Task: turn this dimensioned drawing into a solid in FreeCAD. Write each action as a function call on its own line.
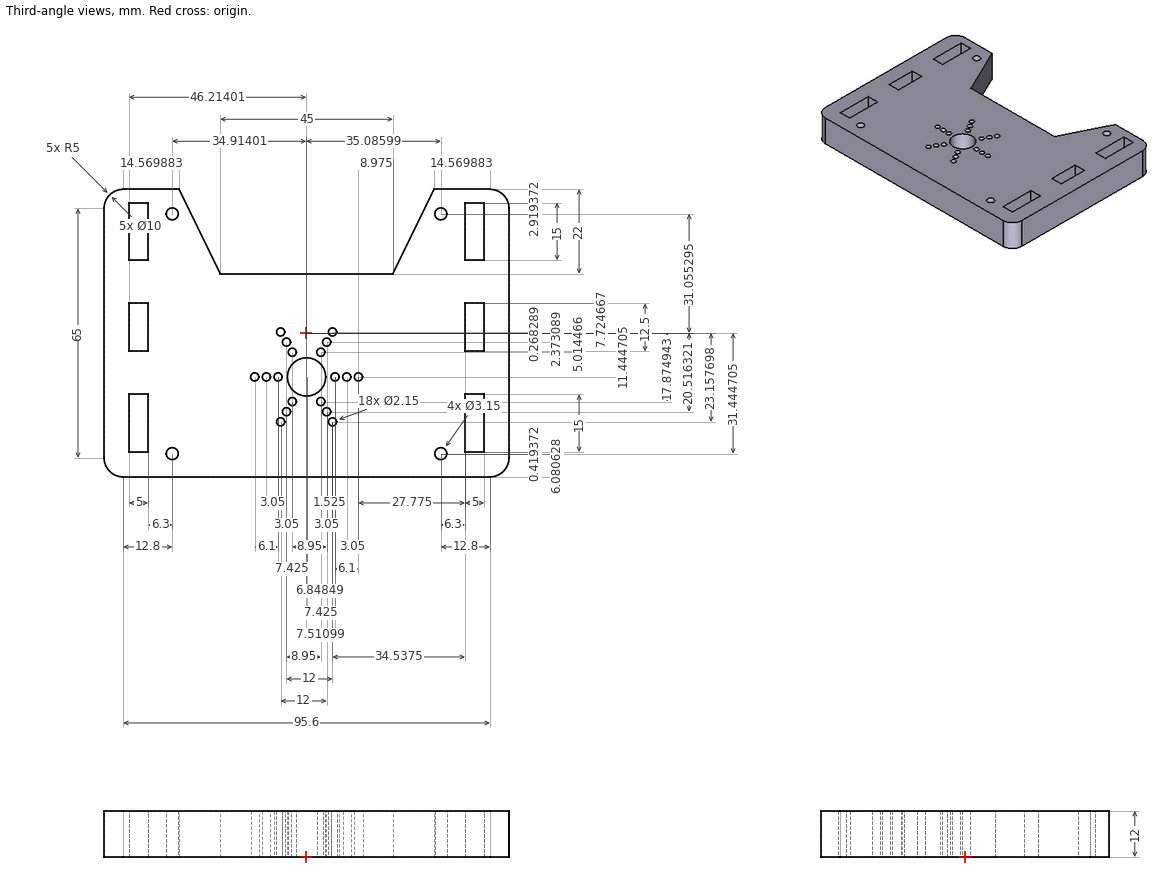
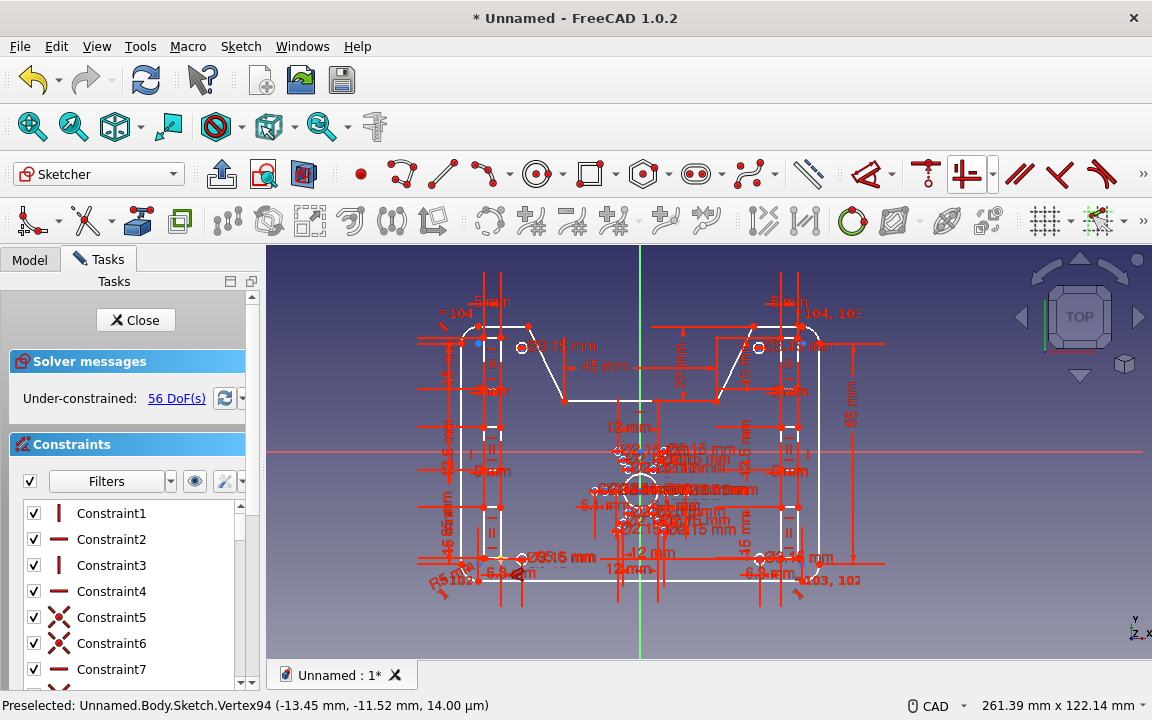
scroll(781, 338, up, 4)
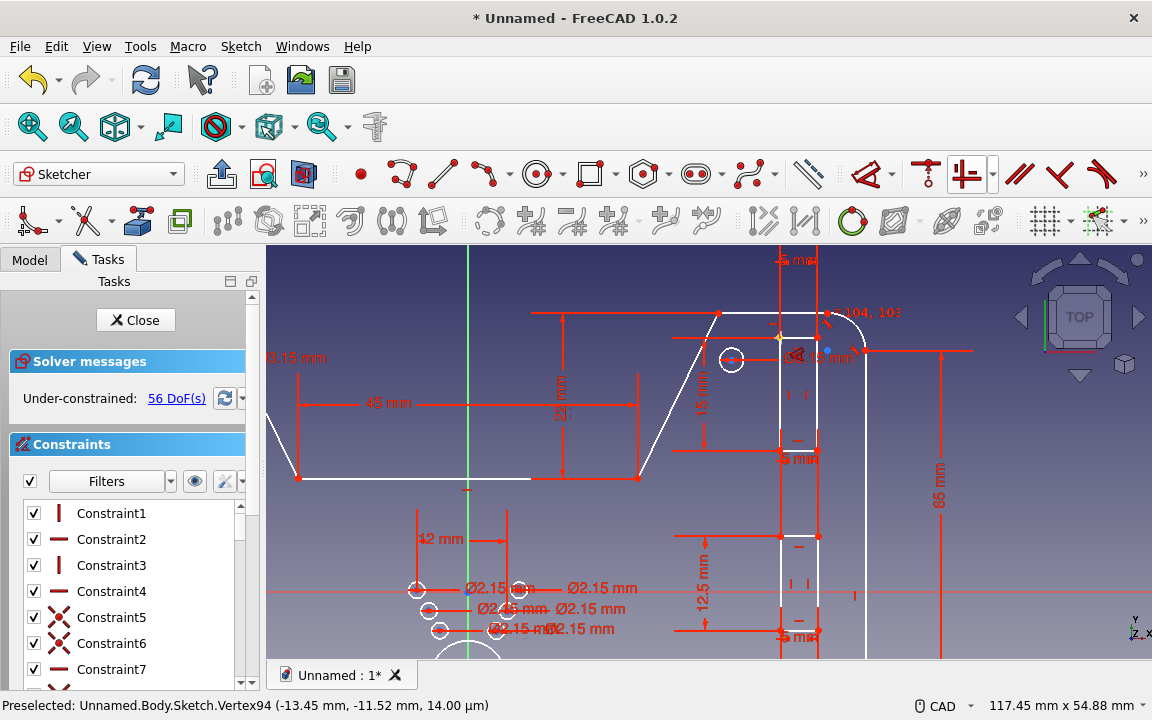
click(780, 338)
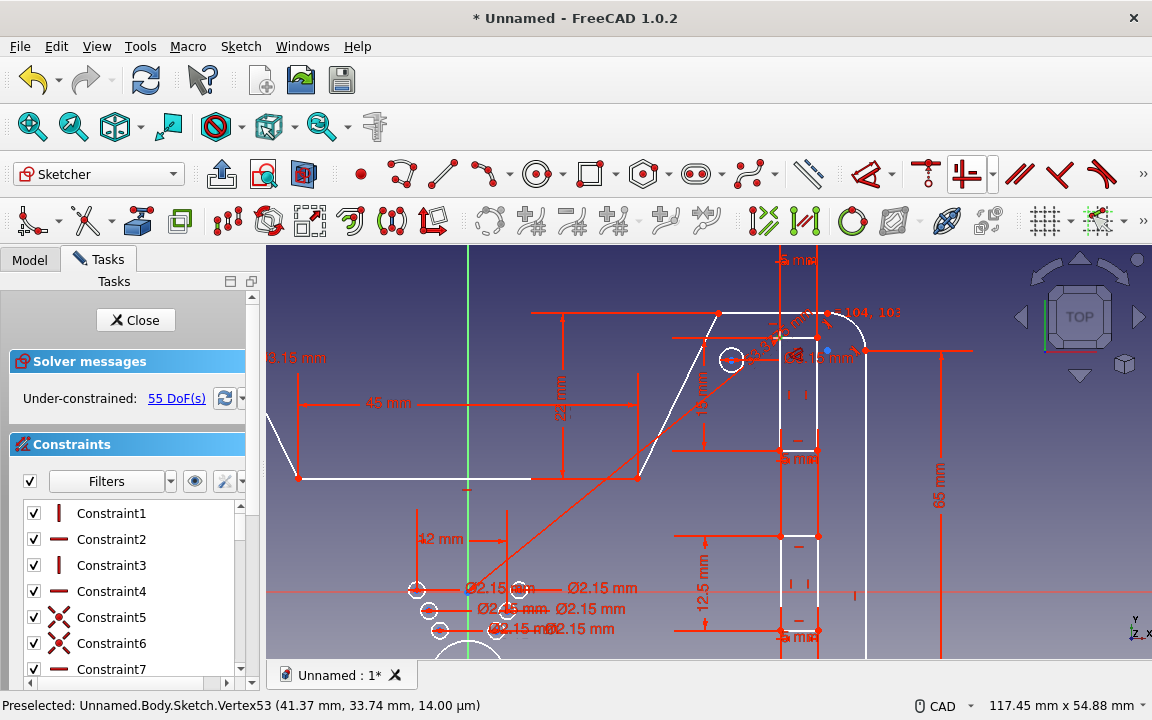
click(732, 360)
click(756, 394)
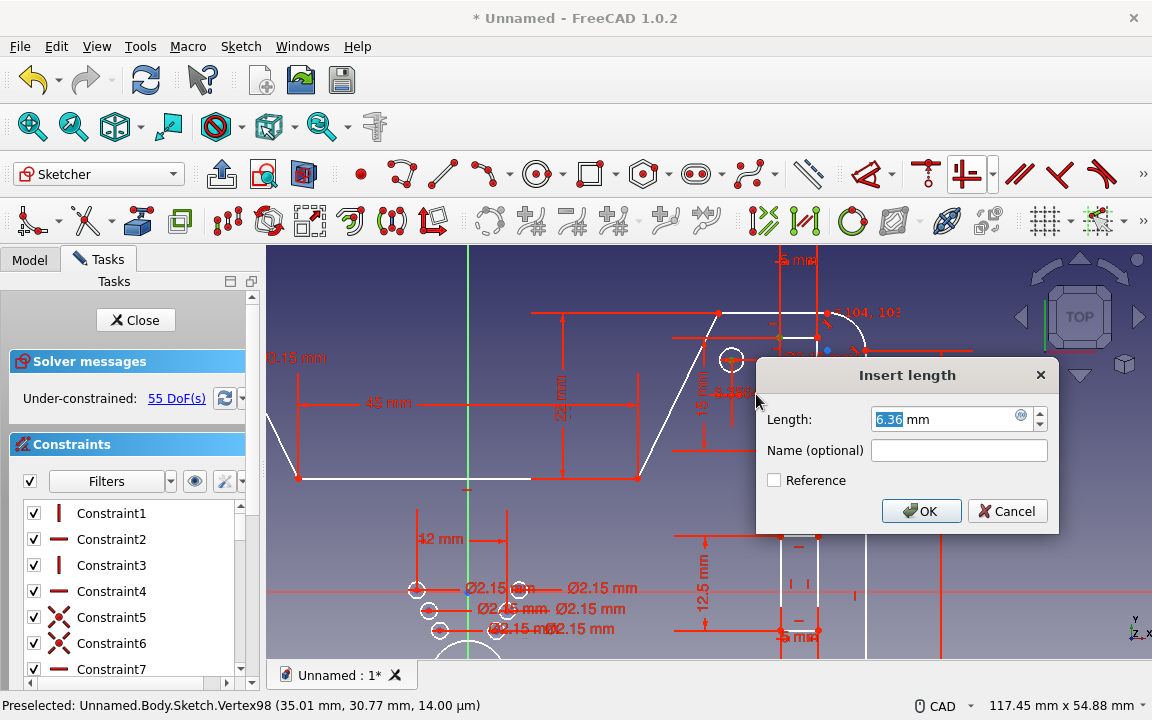
text(6.3)
key(Return)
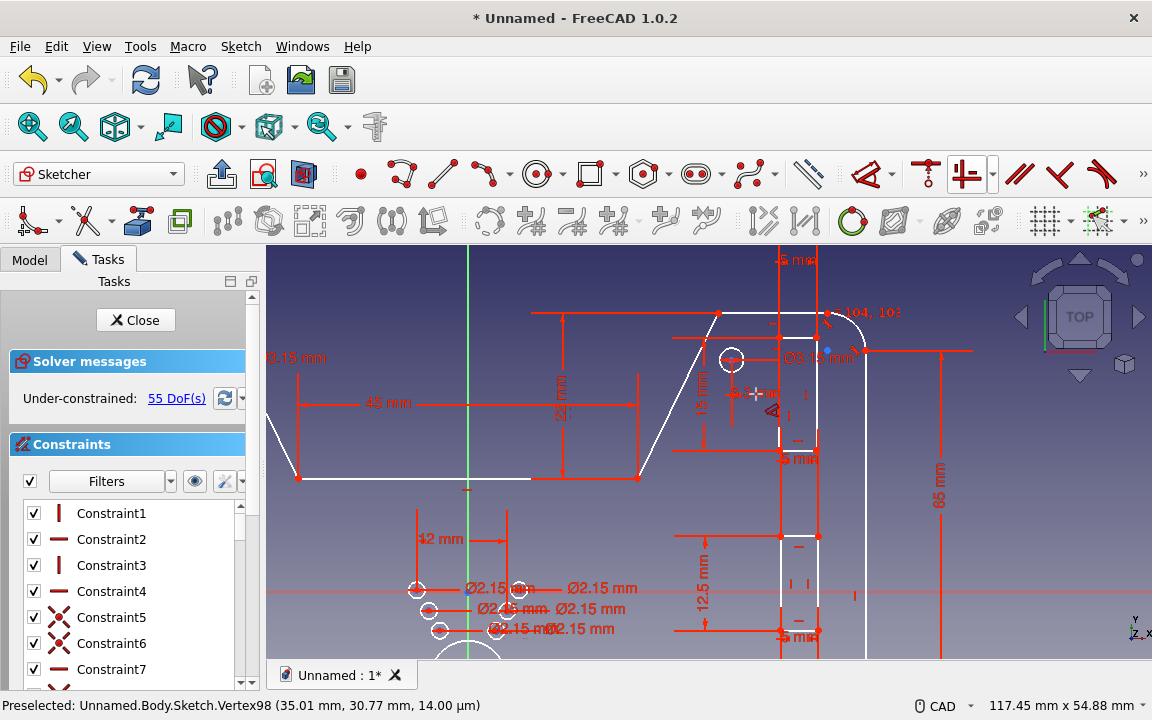
scroll(781, 337, down, 4)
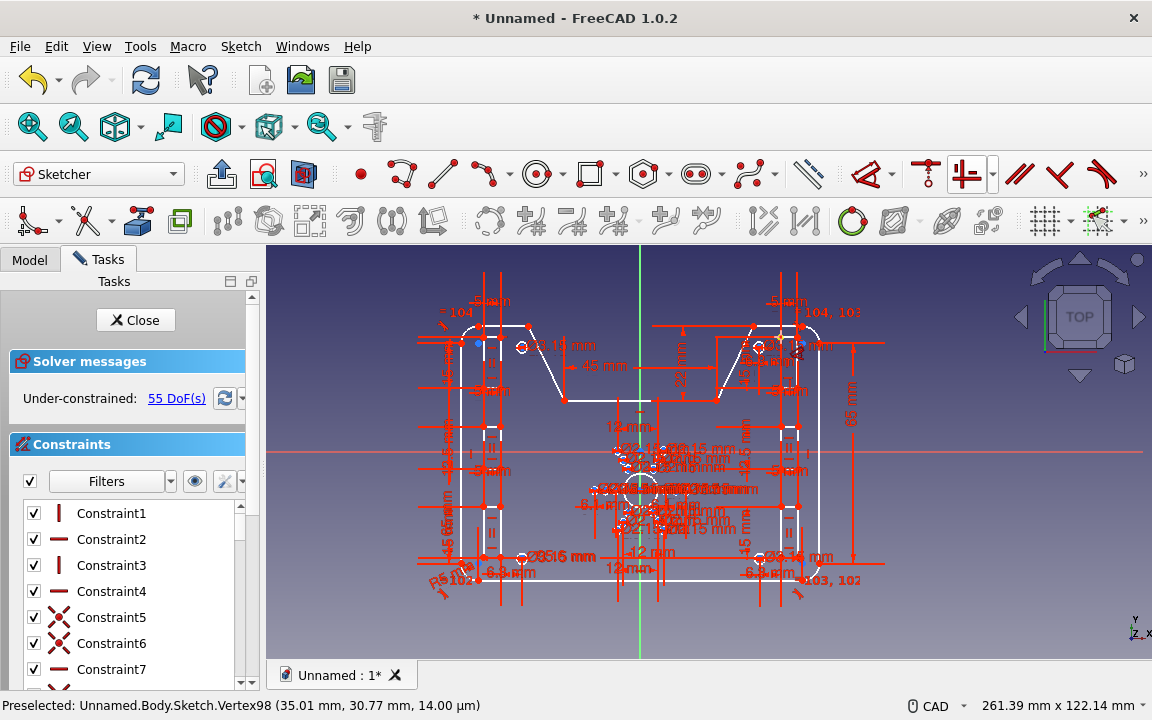
scroll(501, 337, up, 4)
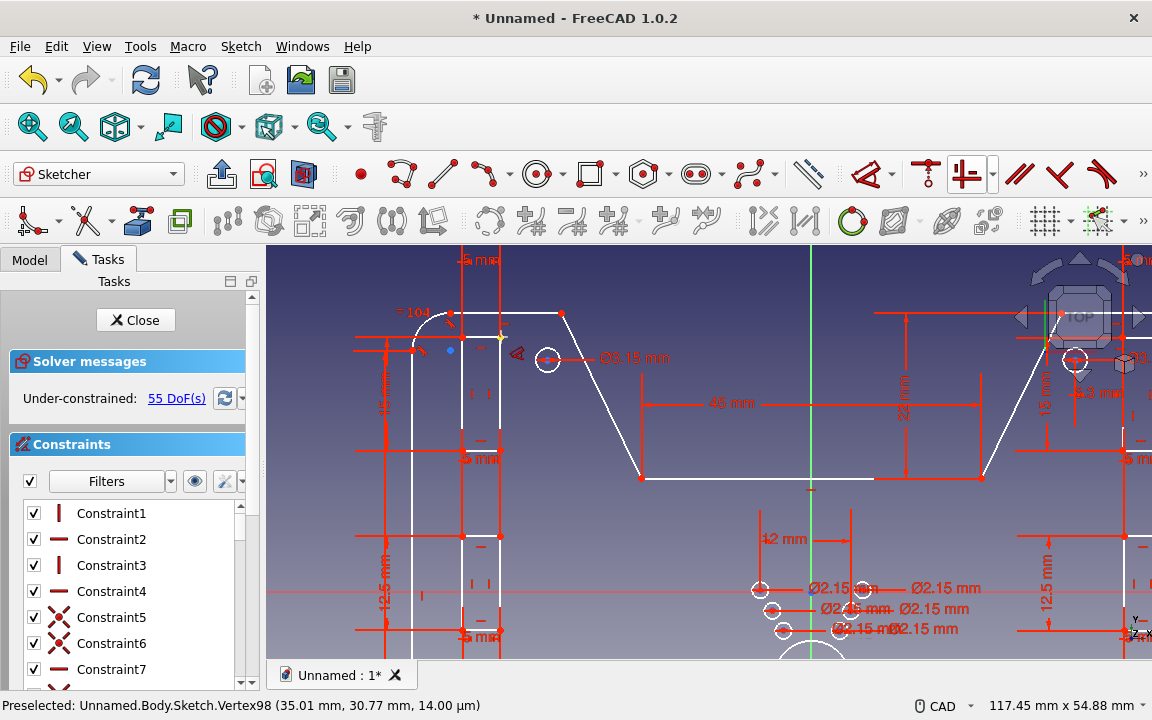
click(500, 337)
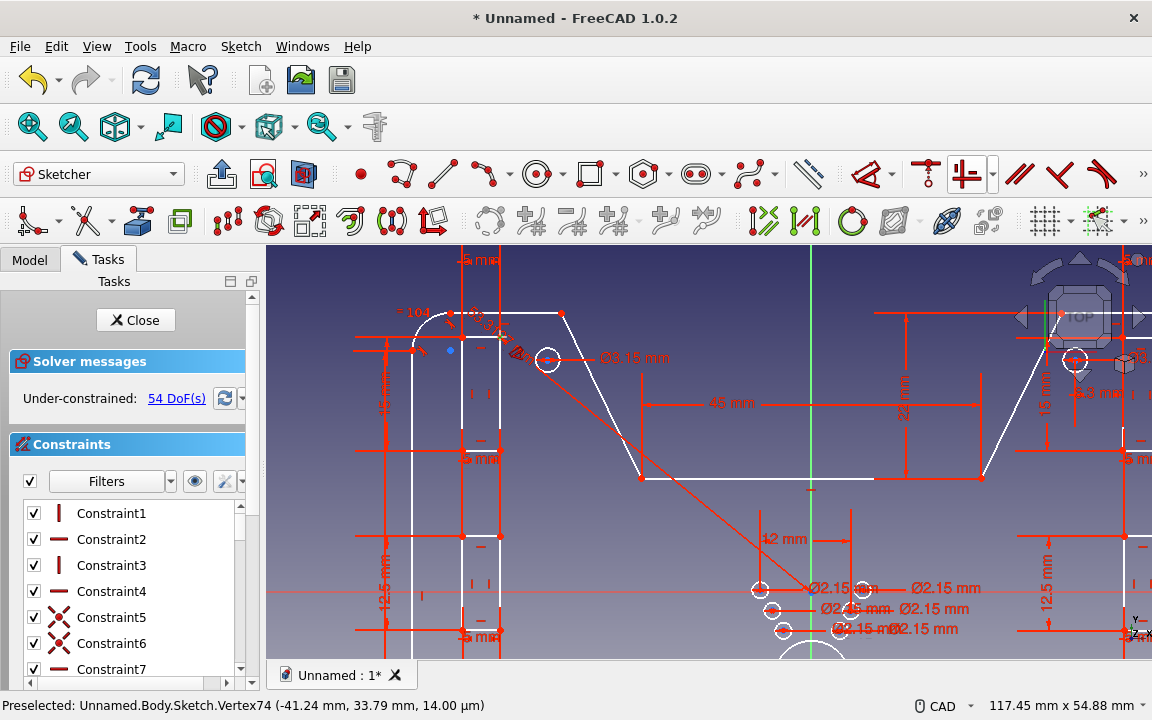
click(548, 360)
click(524, 394)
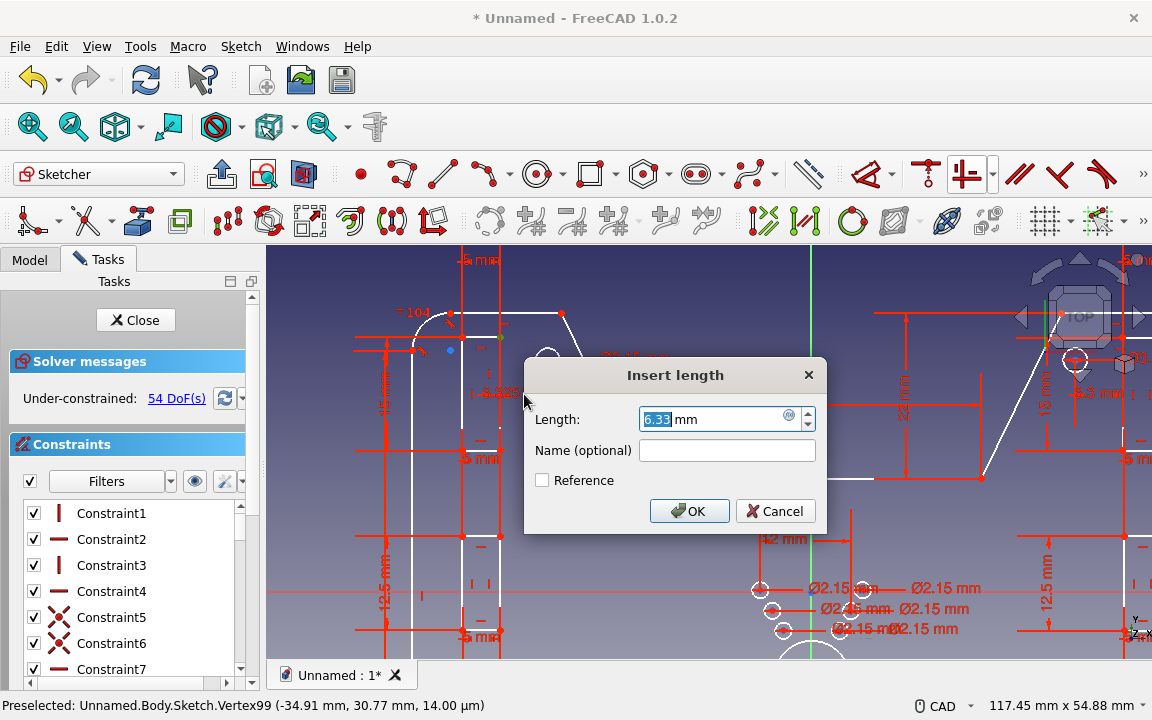
text(6.3)
key(Return)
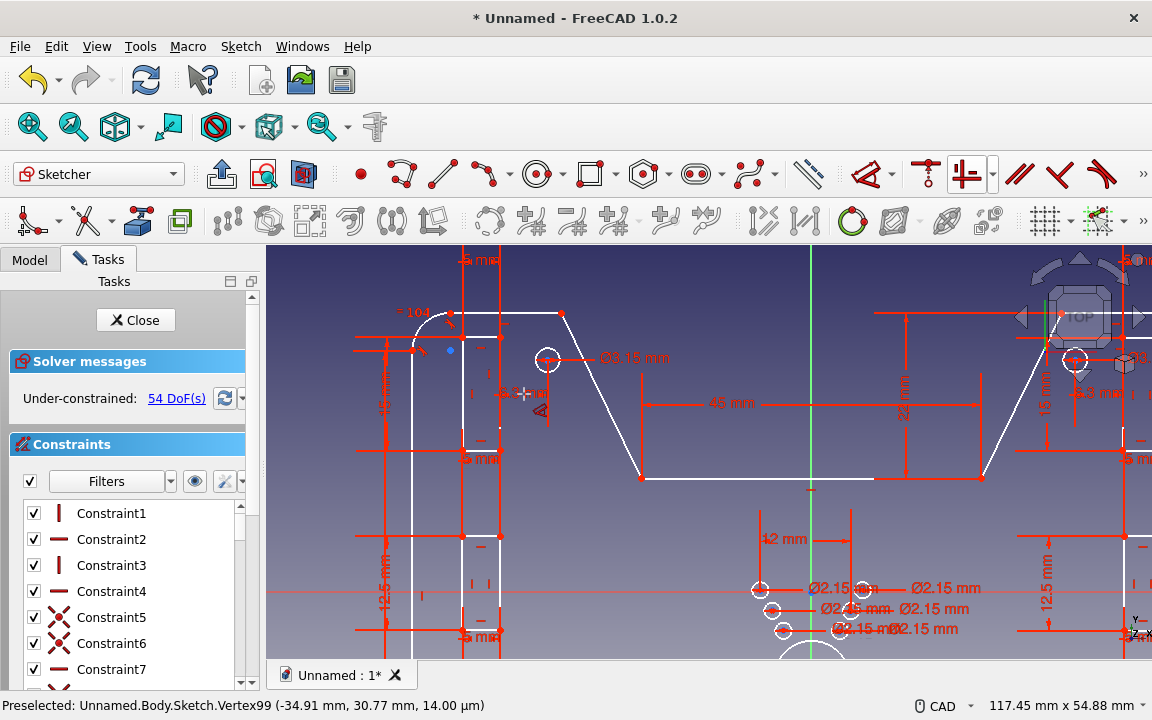
scroll(501, 337, down, 4)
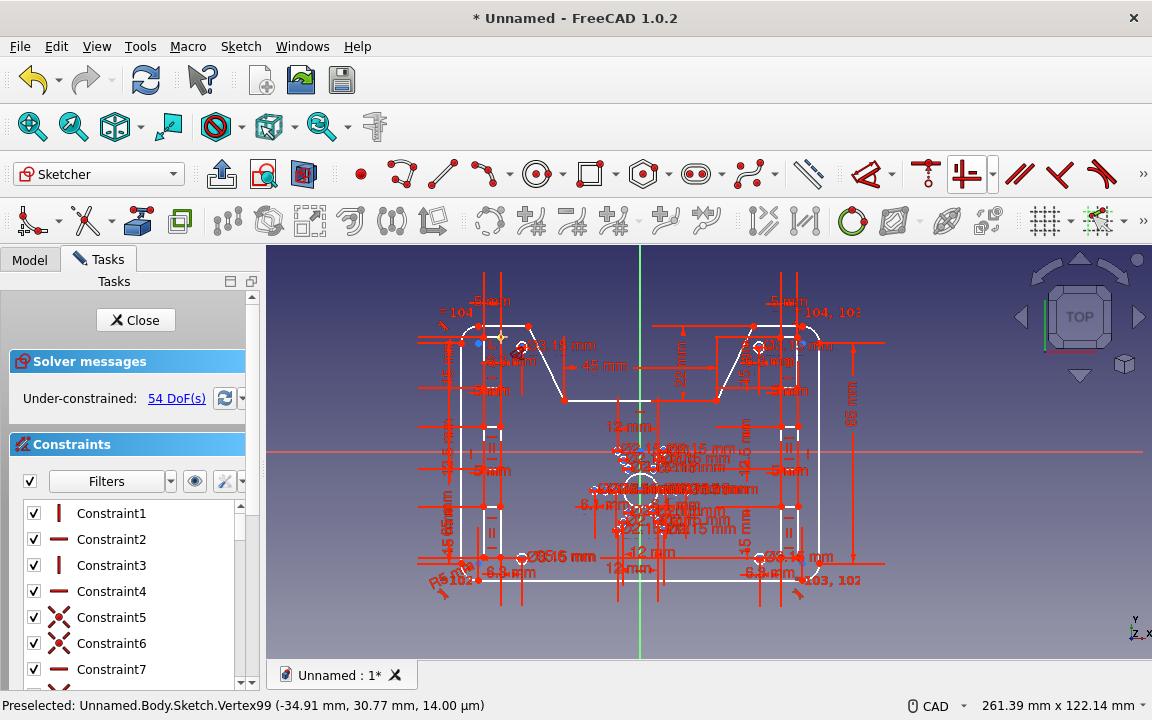
click(802, 581)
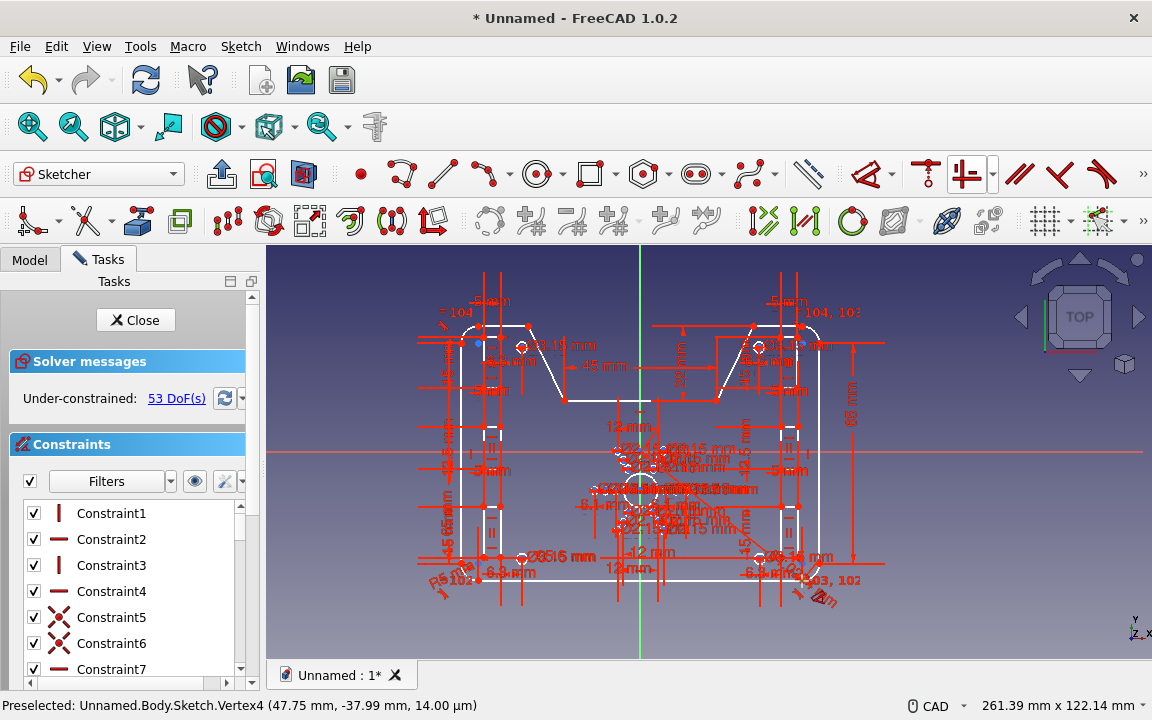
click(760, 559)
click(781, 615)